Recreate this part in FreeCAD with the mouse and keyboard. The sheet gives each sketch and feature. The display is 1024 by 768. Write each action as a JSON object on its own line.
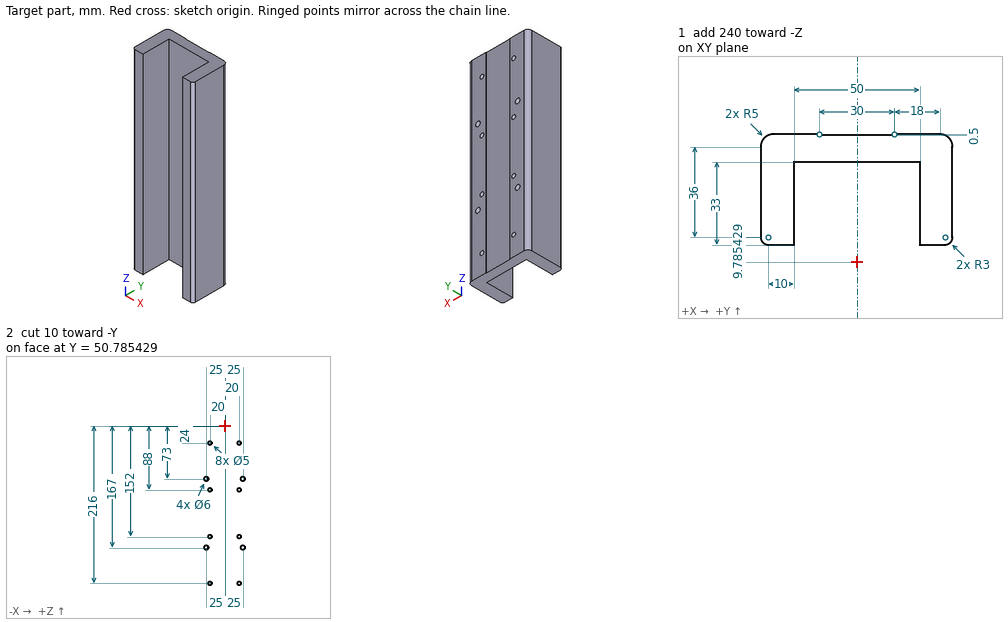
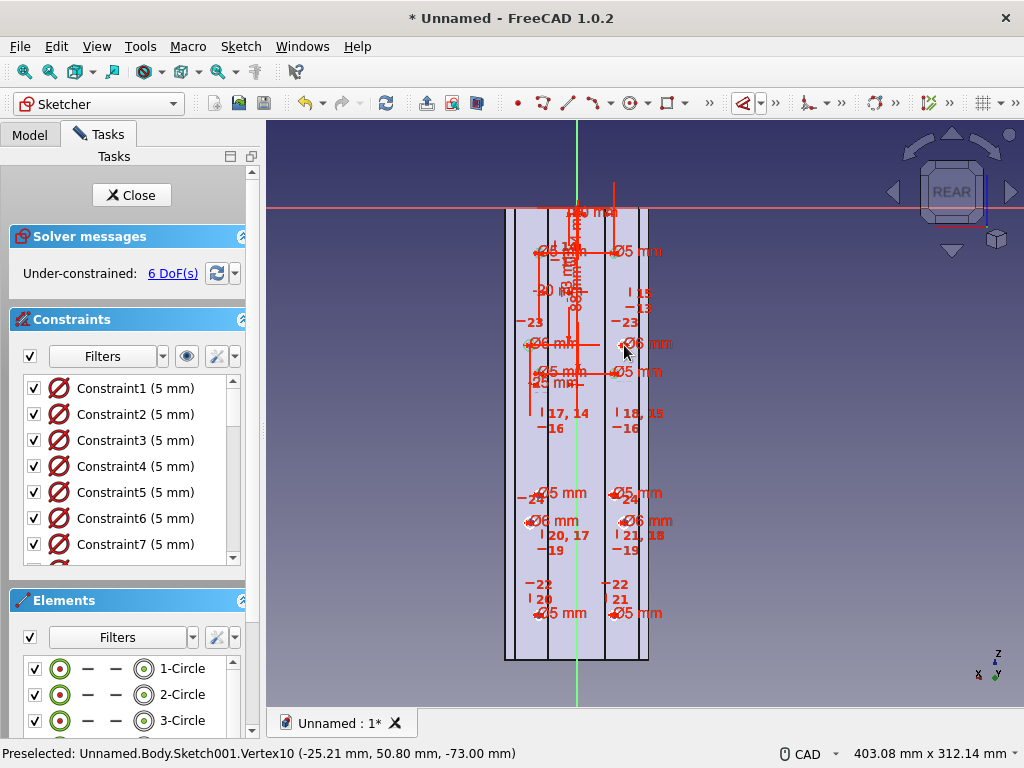
{"action": "key", "text": "l"}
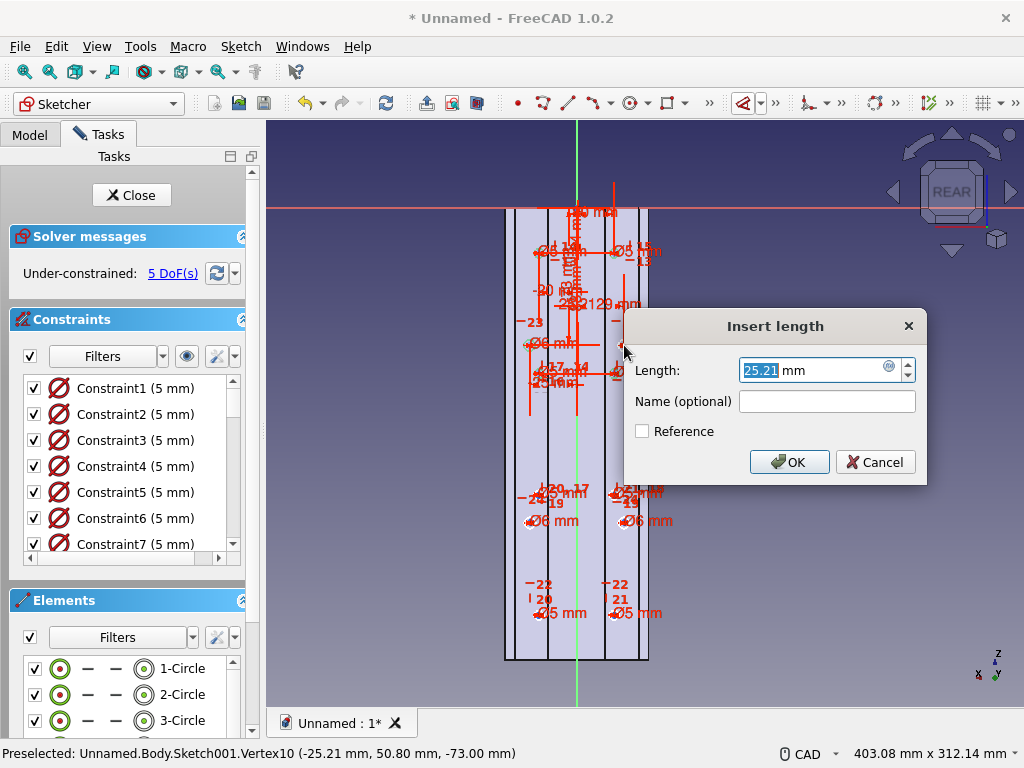
{"action": "type", "text": "25"}
{"action": "key", "text": "Return"}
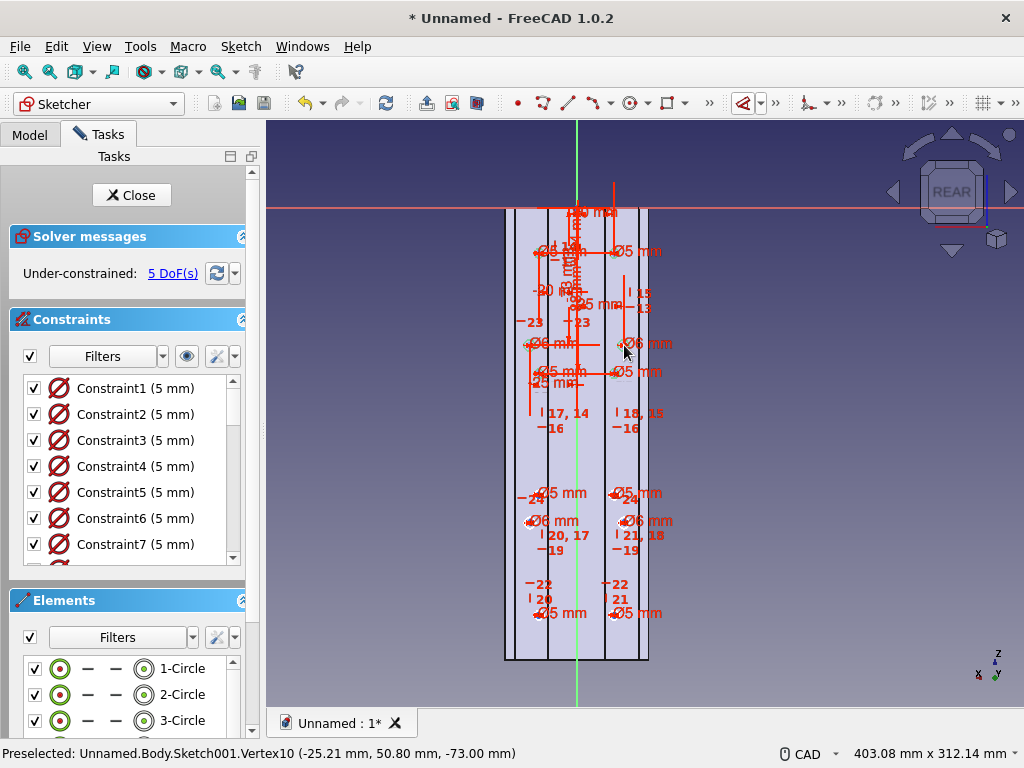
{"action": "left_click", "coordinate": [530, 523]}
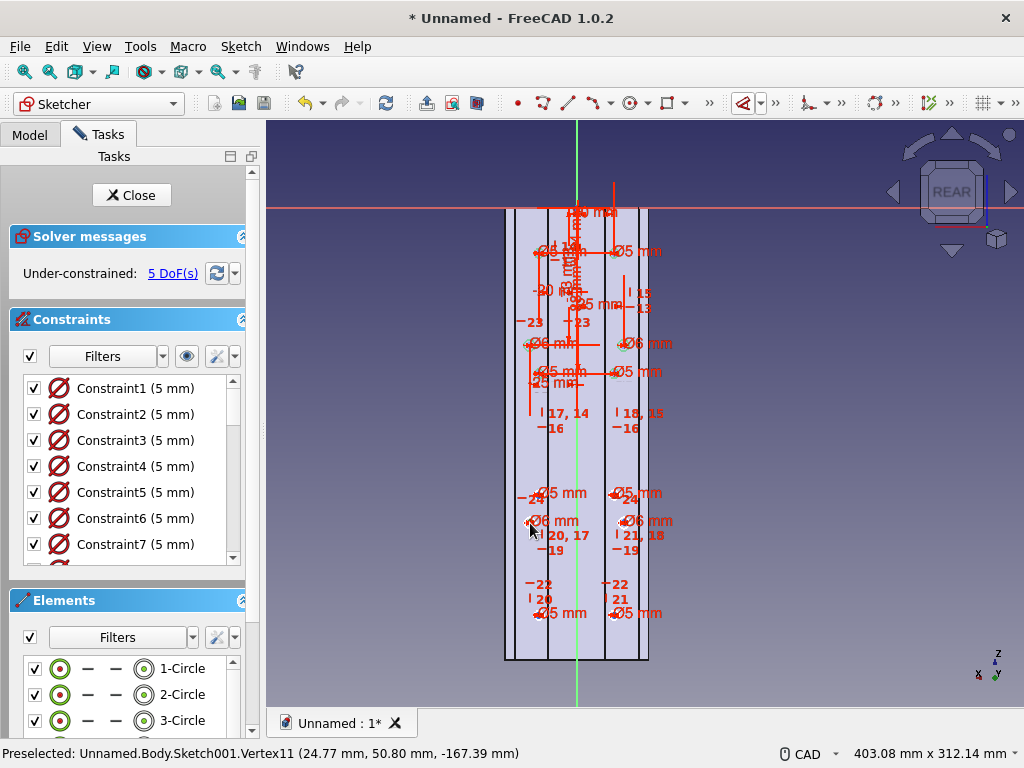
{"action": "key", "text": "l"}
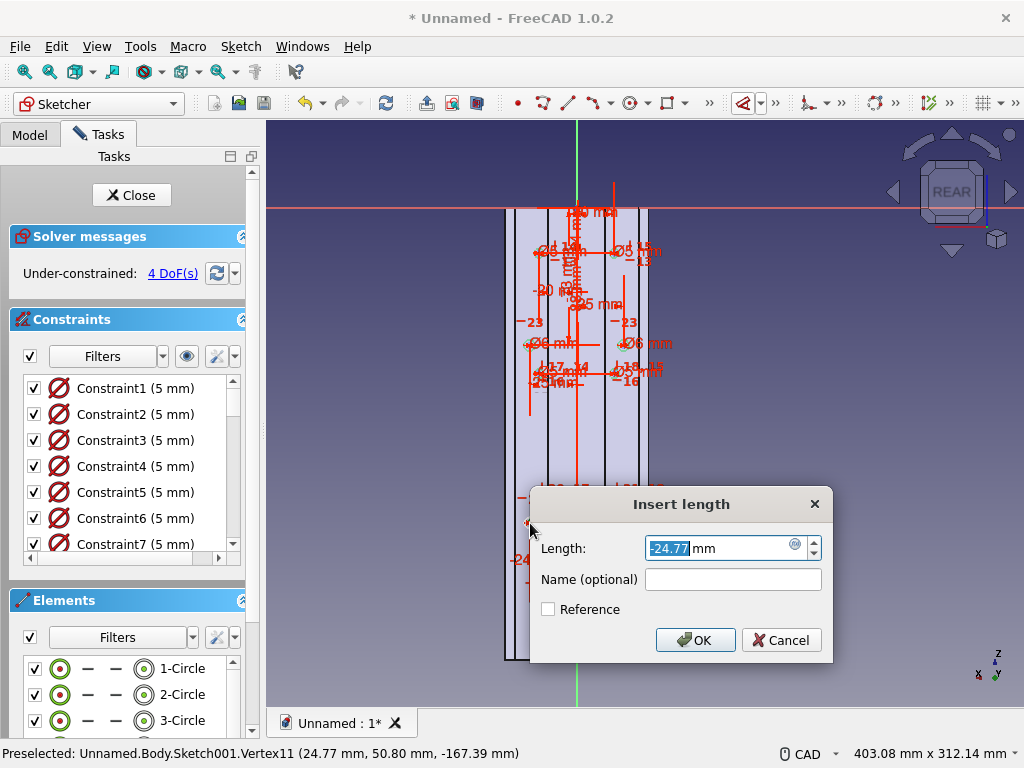
{"action": "type", "text": "-25"}
{"action": "key", "text": "Return"}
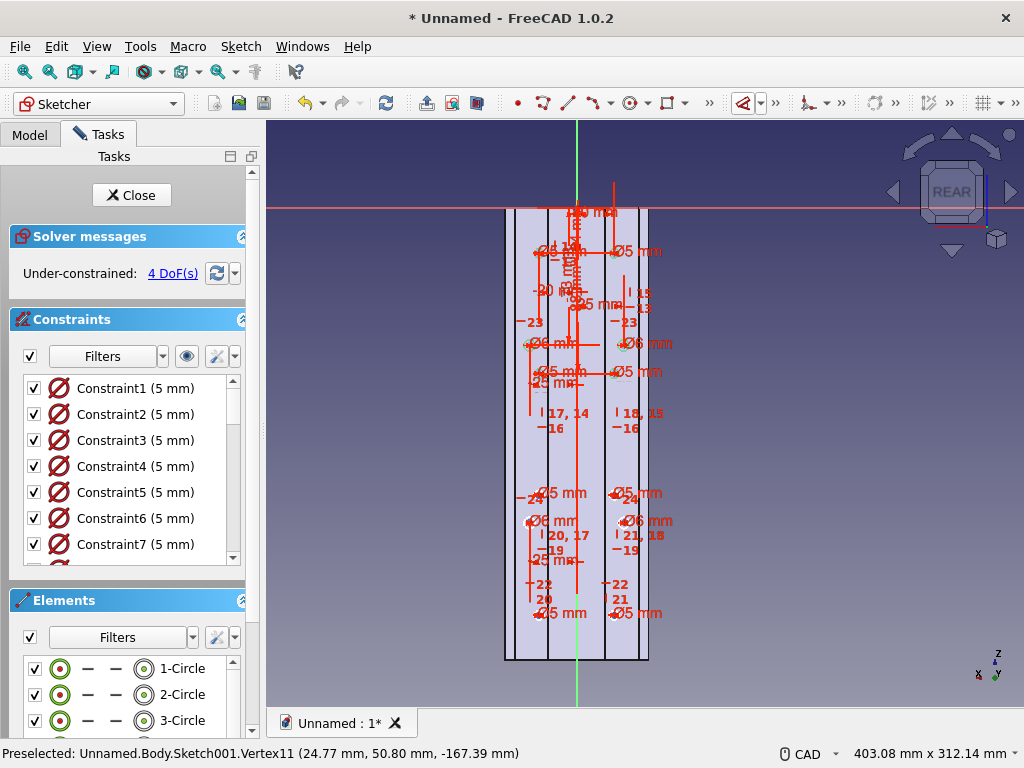
{"action": "left_click", "coordinate": [624, 523]}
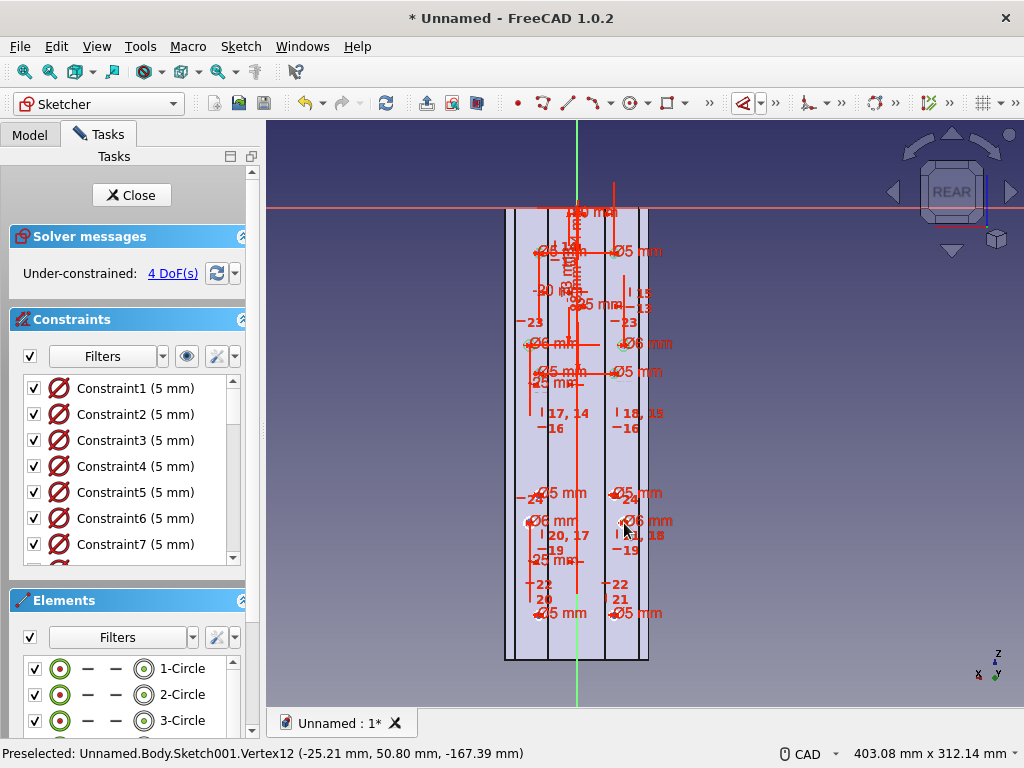
{"action": "left_click", "coordinate": [760, 104]}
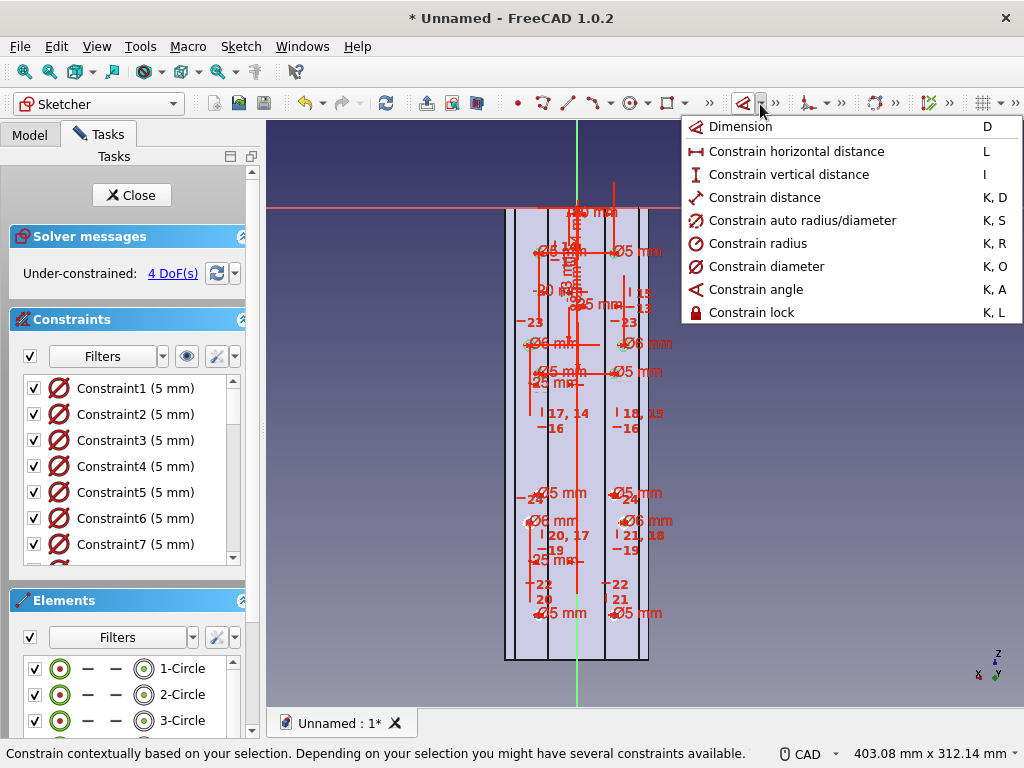
{"action": "left_click", "coordinate": [852, 152]}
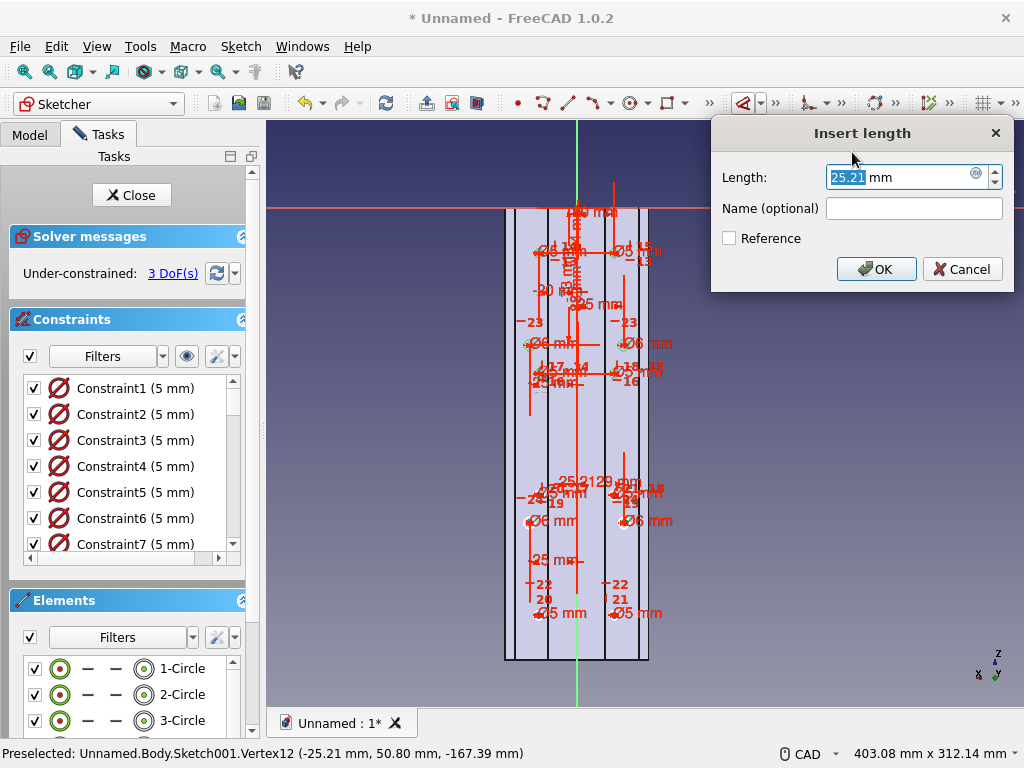
{"action": "type", "text": "25"}
{"action": "key", "text": "Return"}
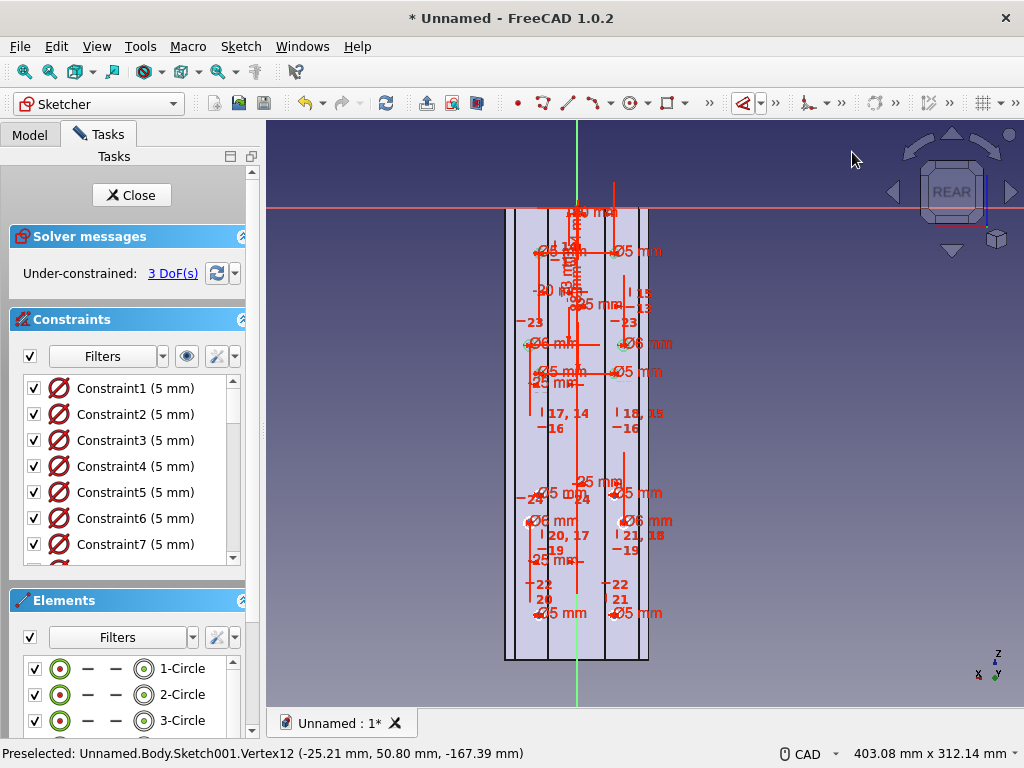
{"action": "left_click", "coordinate": [539, 495]}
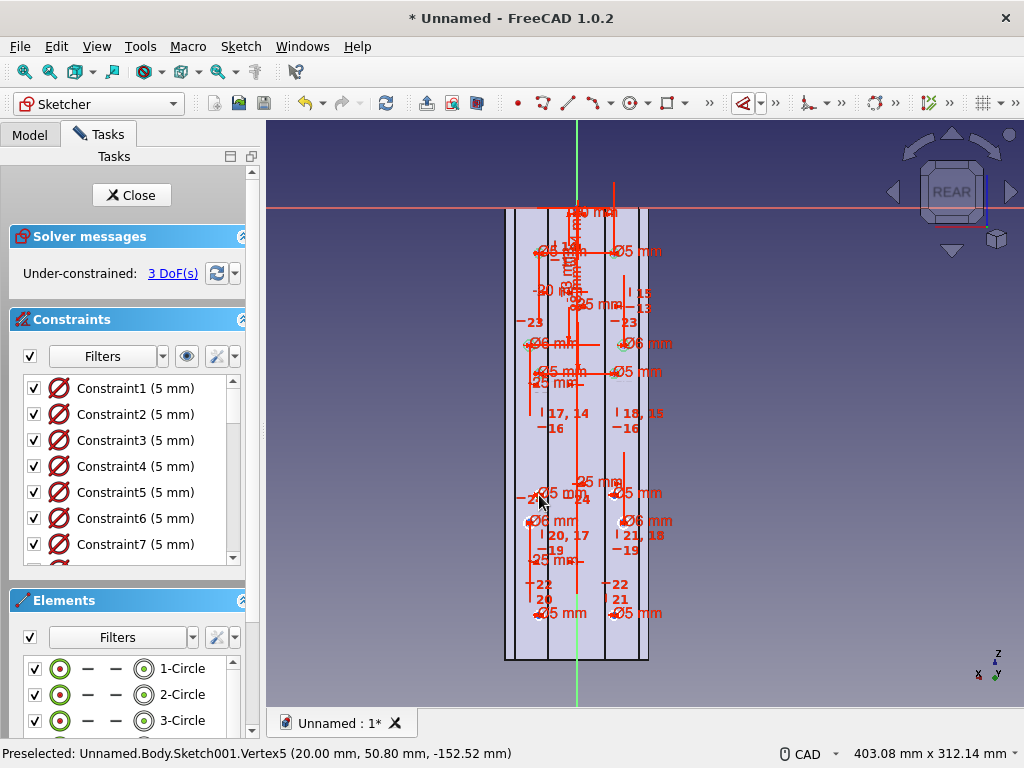
{"action": "key", "text": "i"}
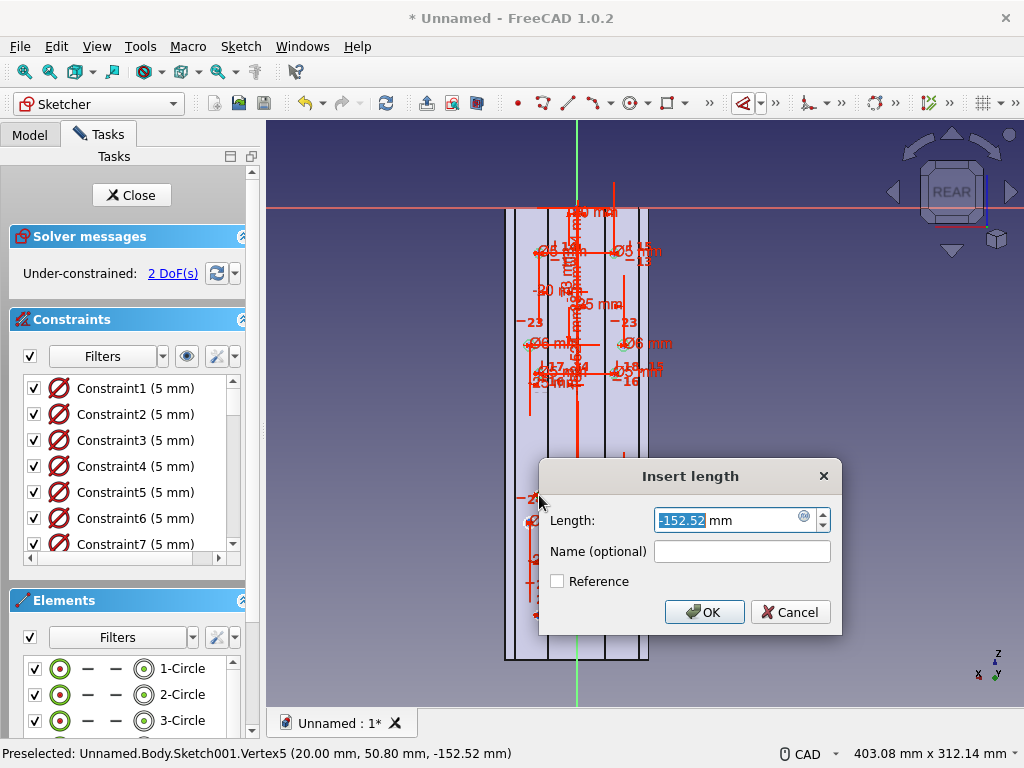
{"action": "type", "text": "-152"}
{"action": "key", "text": "Return"}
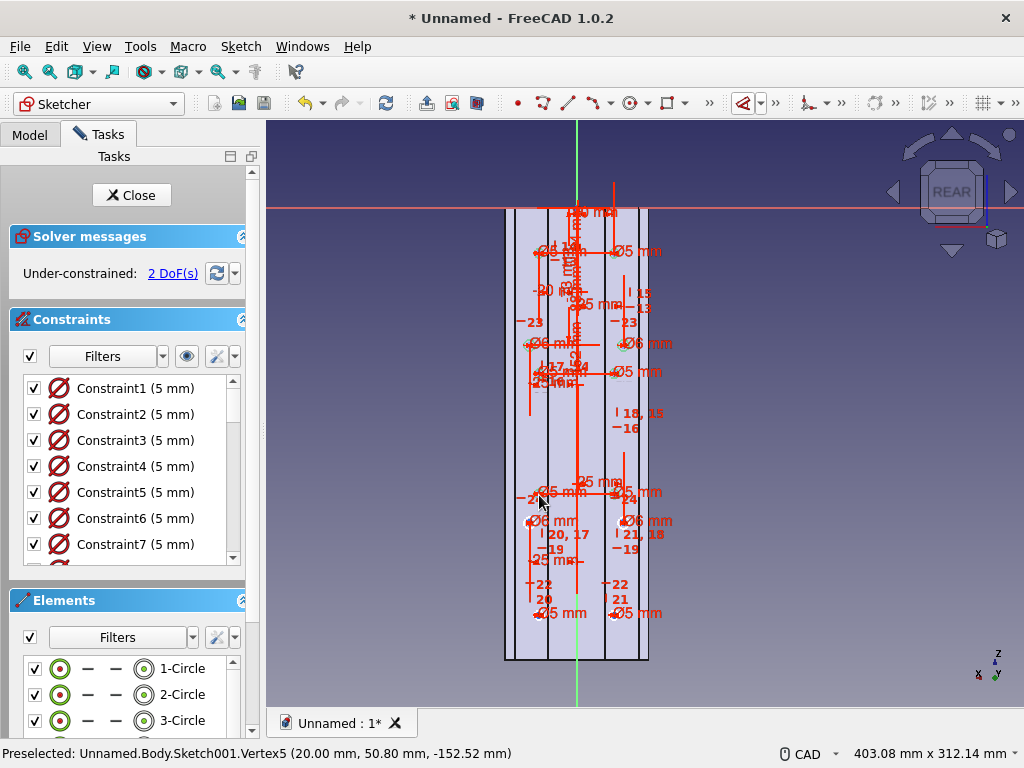
{"action": "left_click", "coordinate": [539, 615]}